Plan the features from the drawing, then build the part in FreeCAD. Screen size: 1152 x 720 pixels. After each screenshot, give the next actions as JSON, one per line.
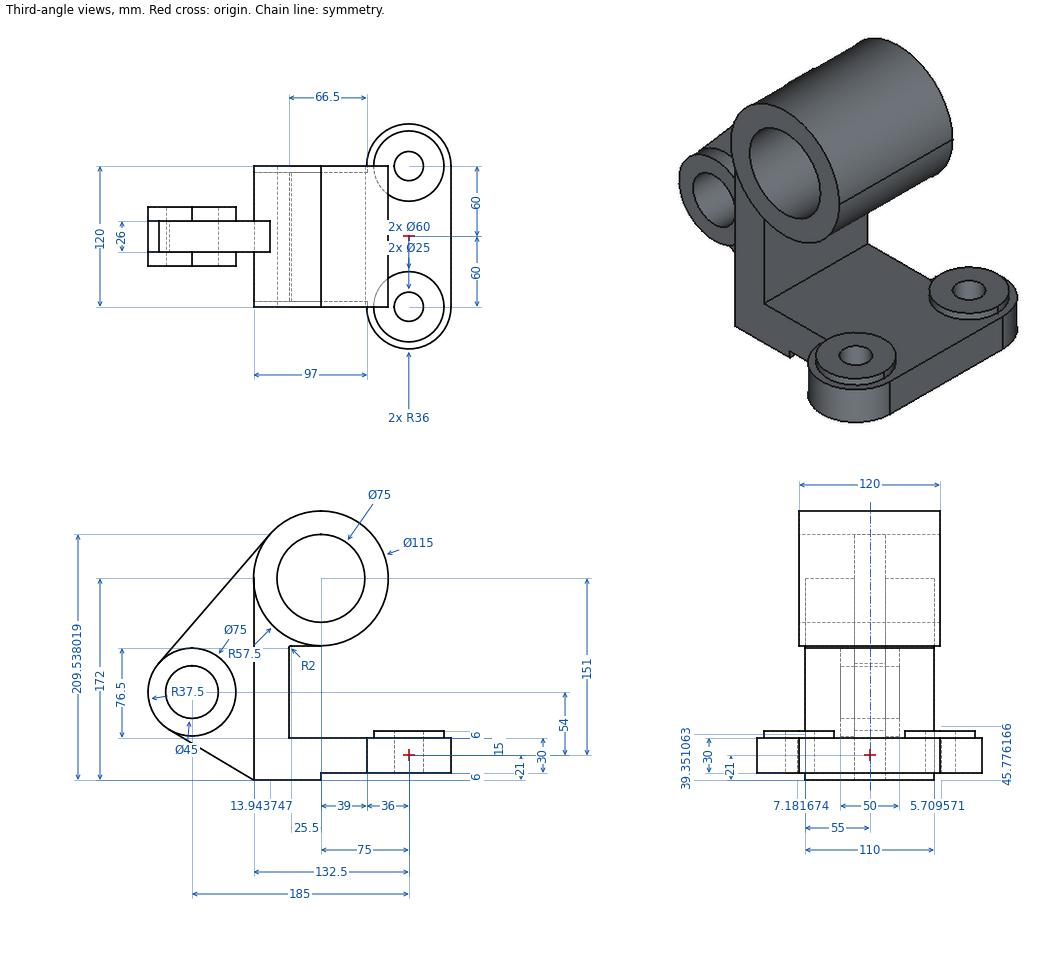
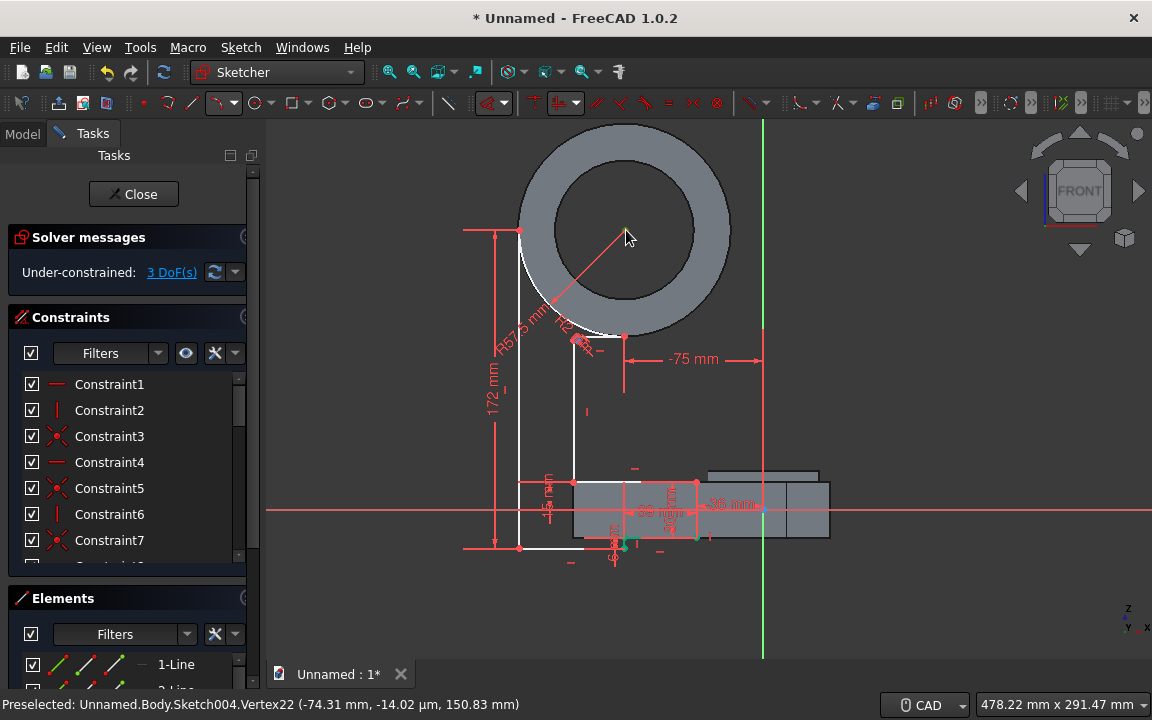
{"action": "key", "text": "l"}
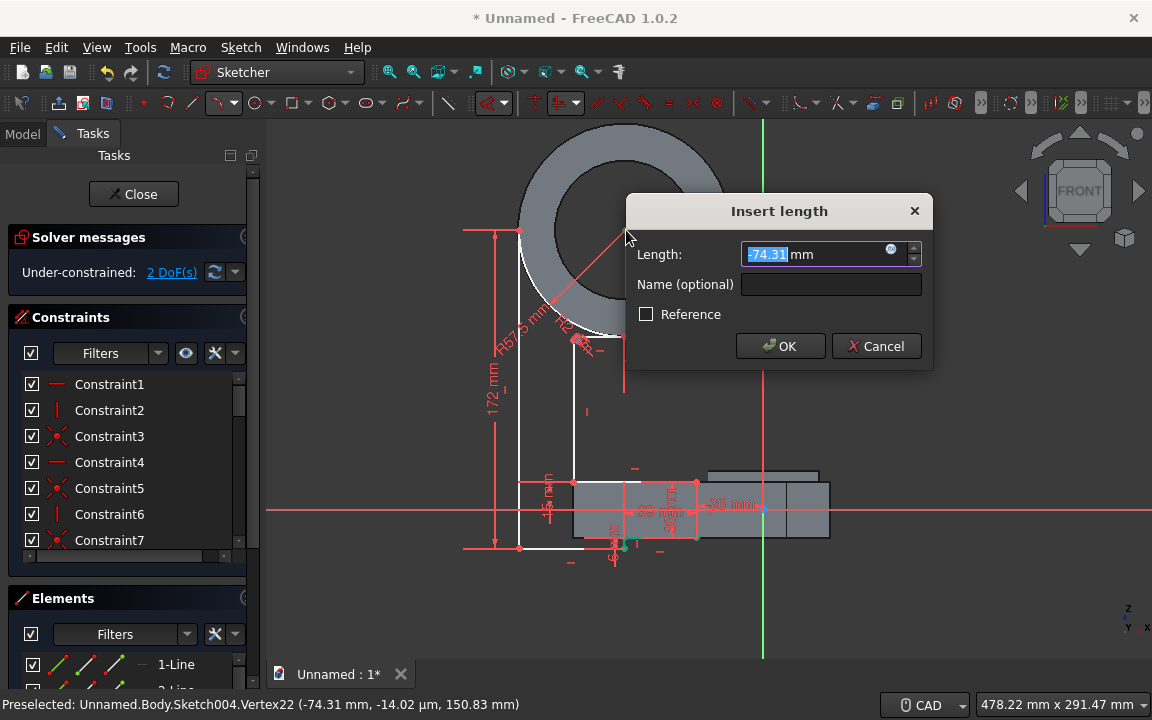
{"action": "type", "text": "-75"}
{"action": "key", "text": "Return"}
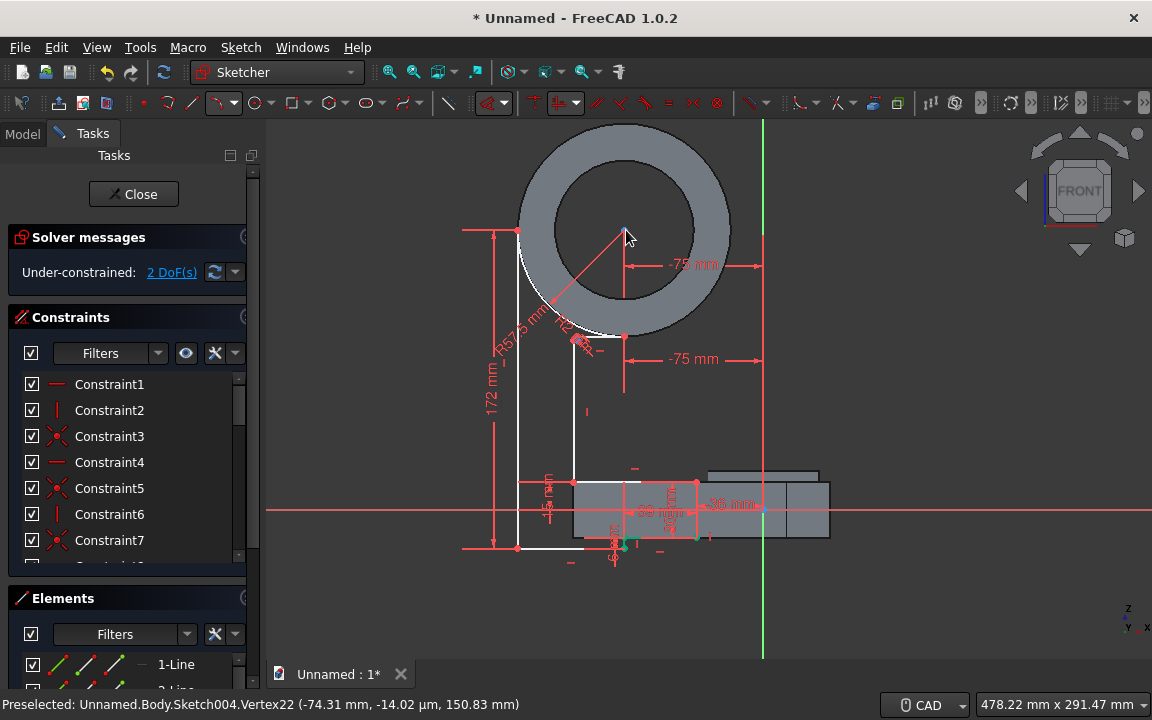
{"action": "scroll", "coordinate": [587, 337], "scroll_direction": "up", "scroll_amount": 4}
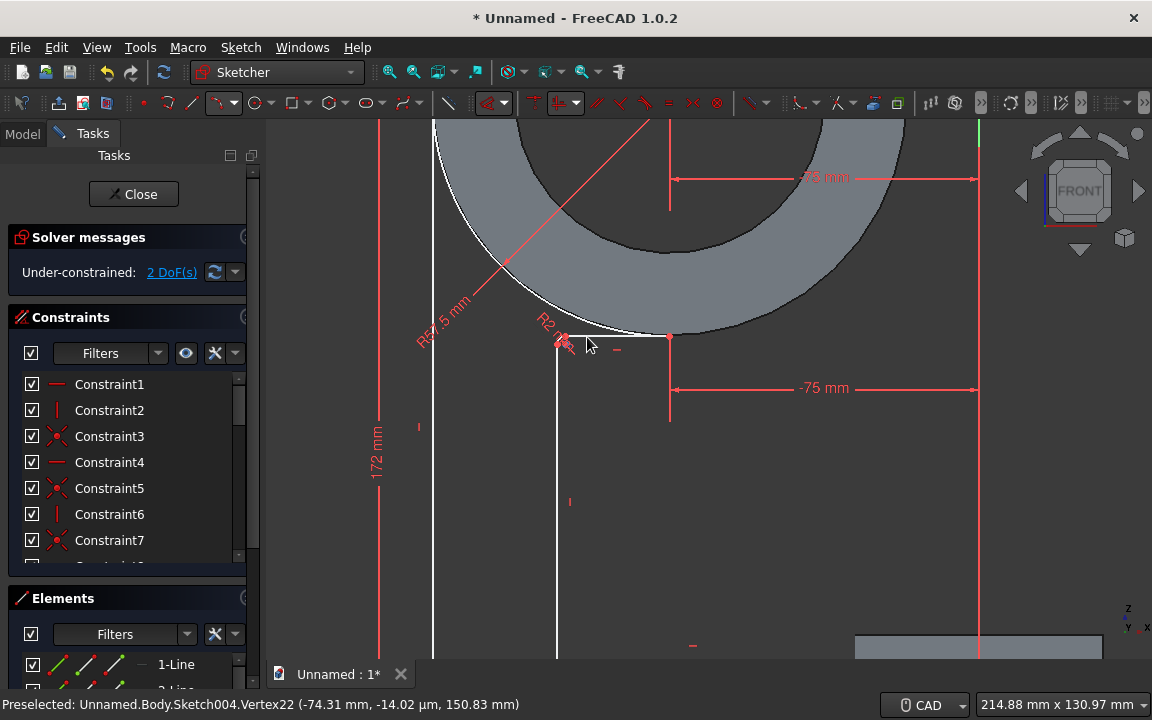
{"action": "left_click", "coordinate": [586, 336]}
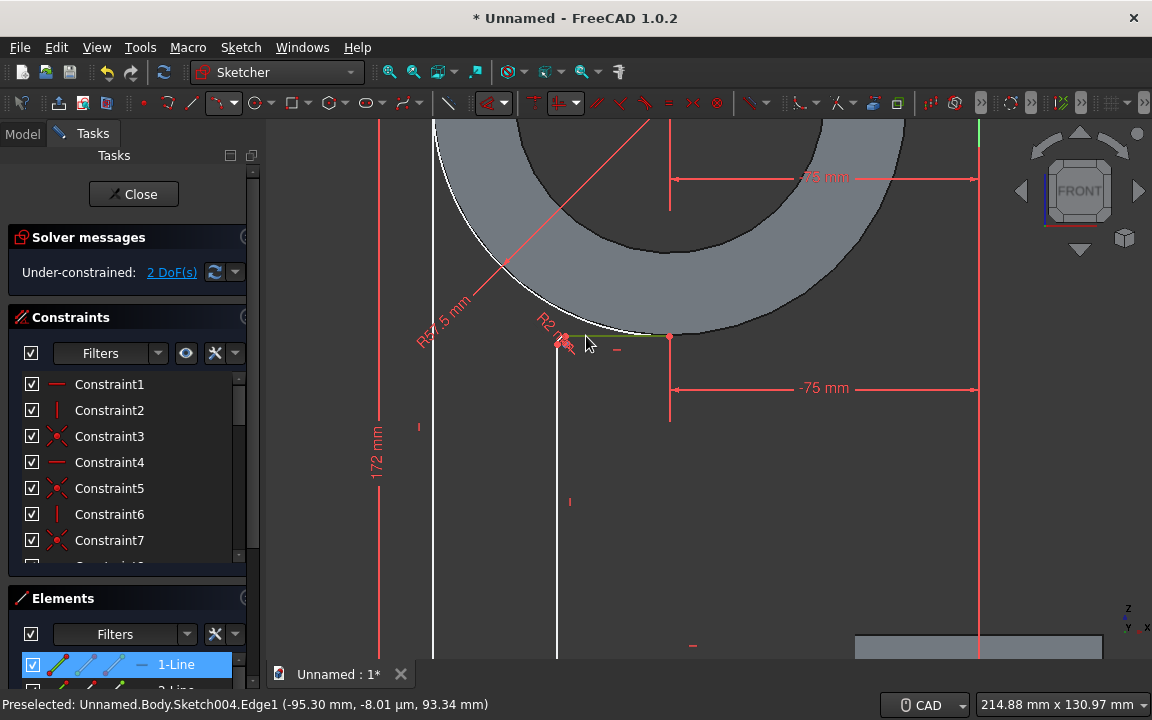
{"action": "key", "text": "l"}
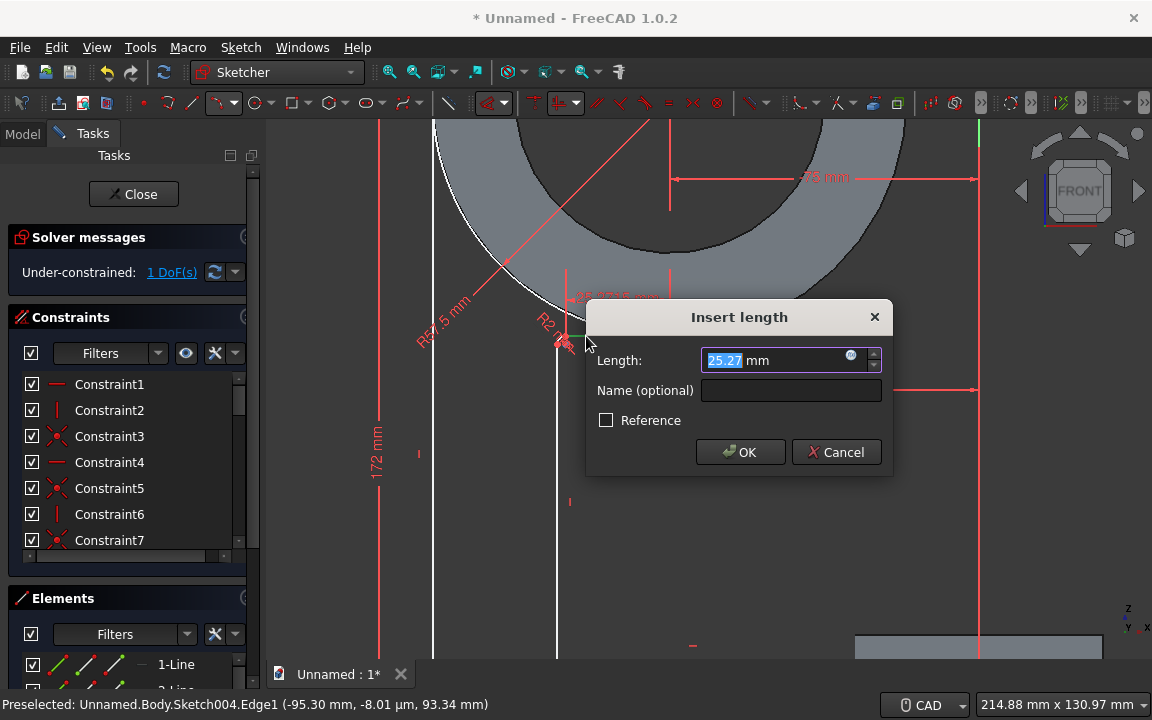
{"action": "type", "text": "25.5"}
{"action": "key", "text": "Return"}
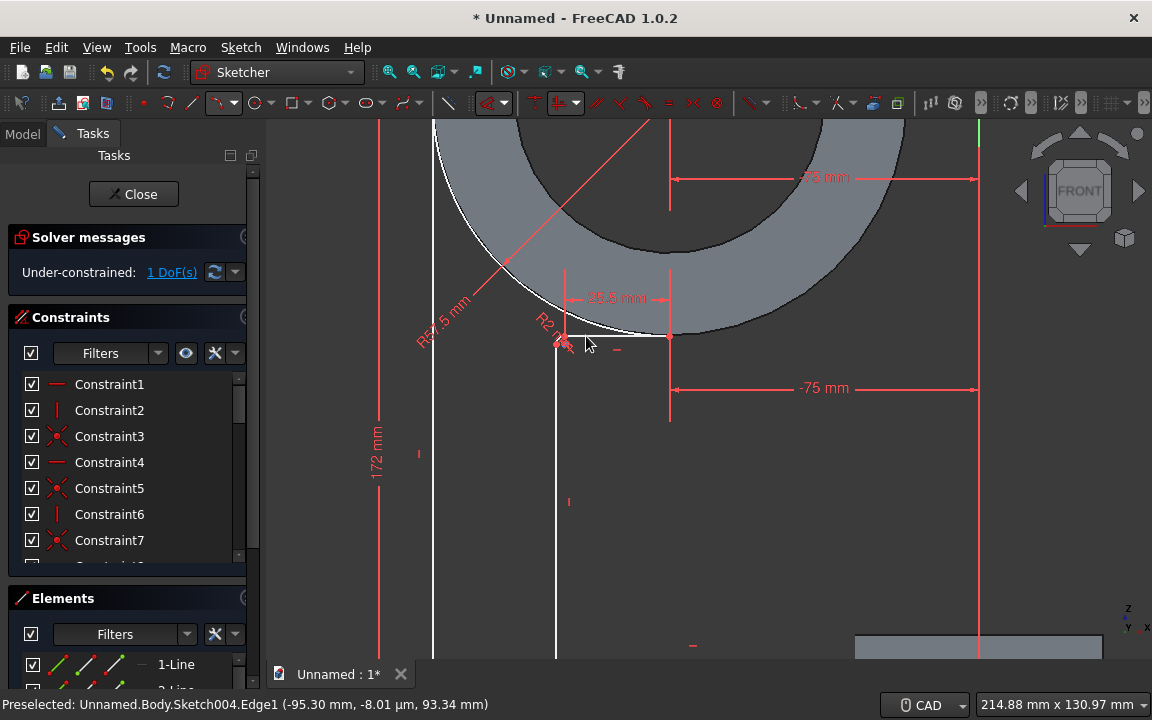
{"action": "left_click", "coordinate": [556, 439]}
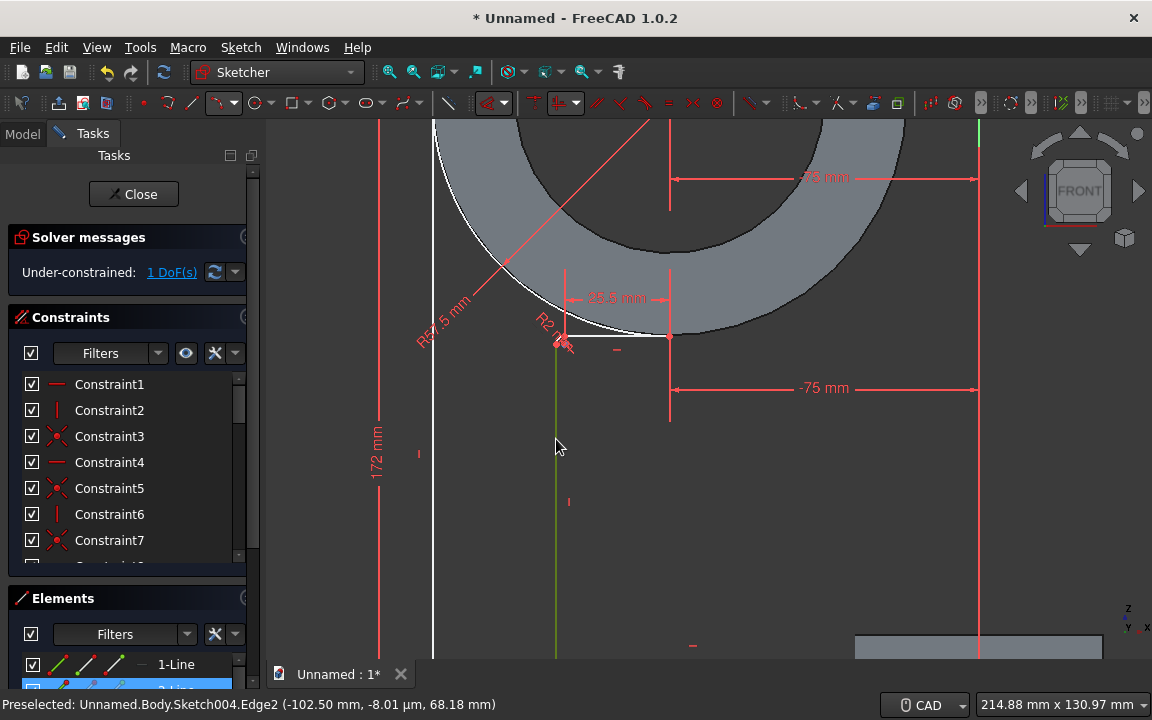
{"action": "key", "text": "i"}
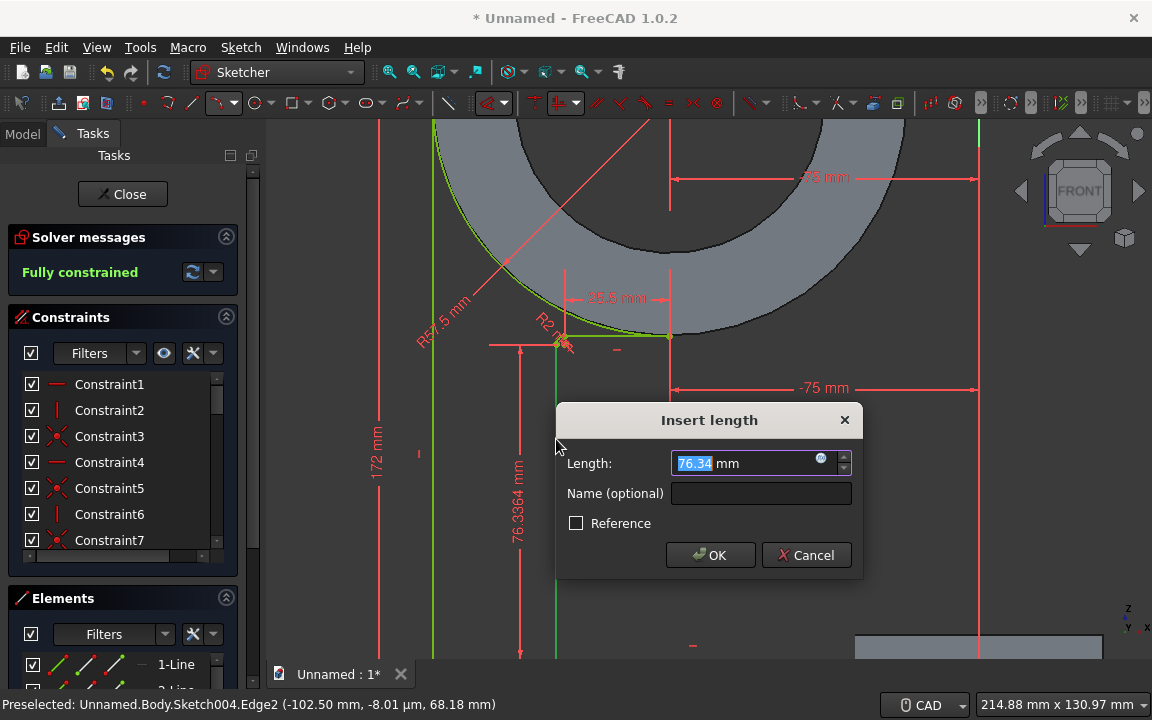
{"action": "type", "text": "76.5"}
{"action": "key", "text": "Return"}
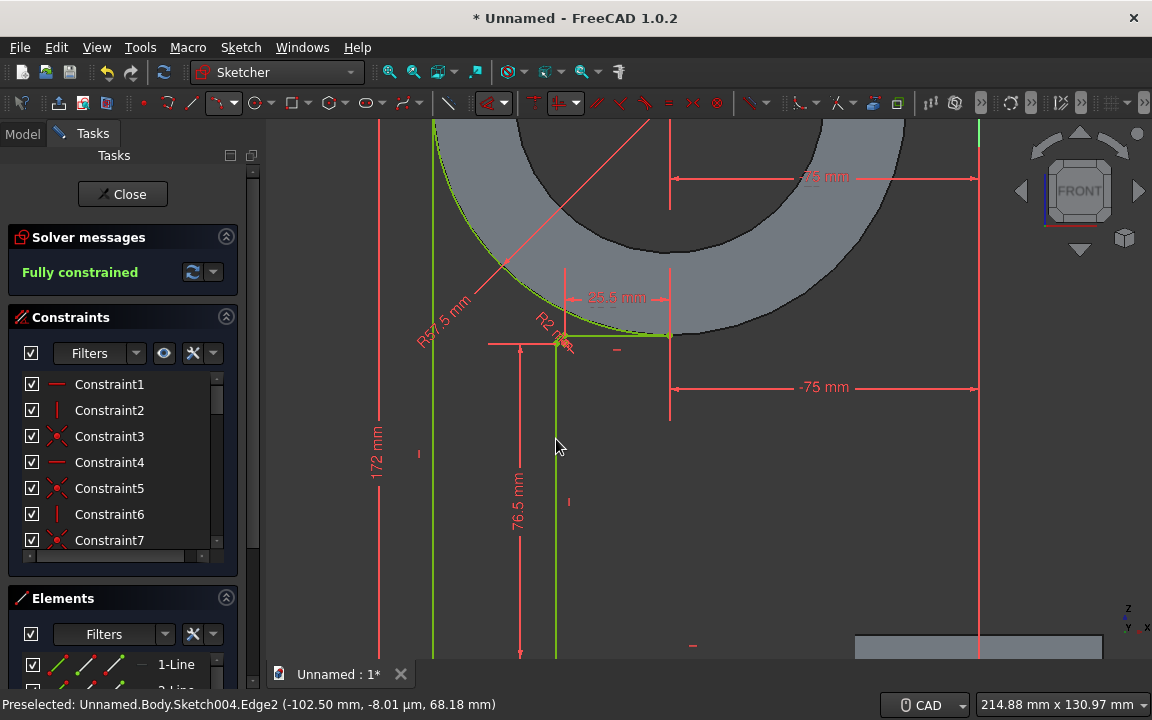
{"action": "left_click", "coordinate": [123, 194]}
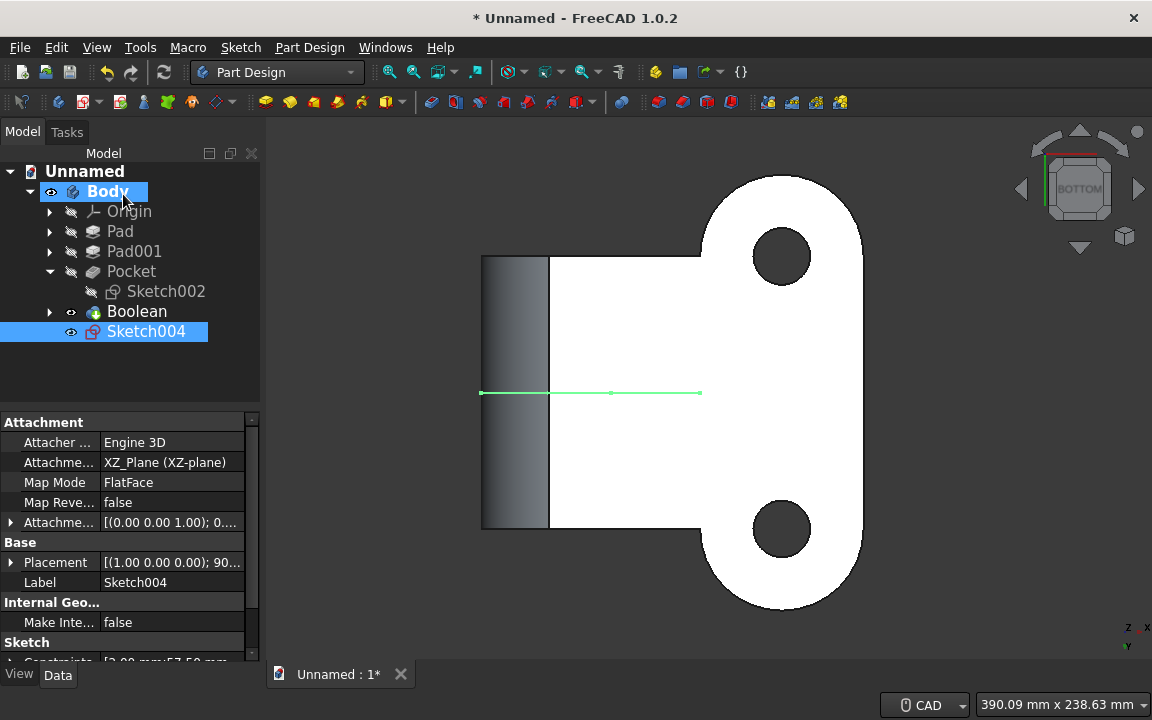
{"action": "left_click", "coordinate": [266, 102]}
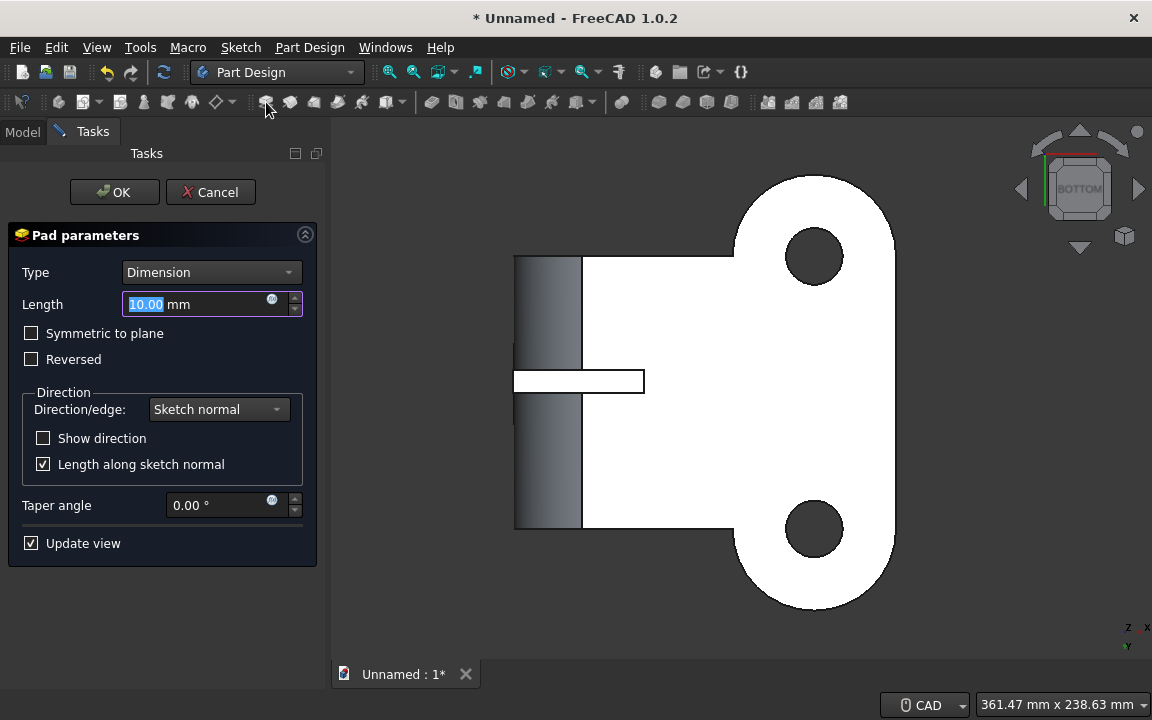
{"action": "type", "text": "110"}
{"action": "key", "text": "Tab"}